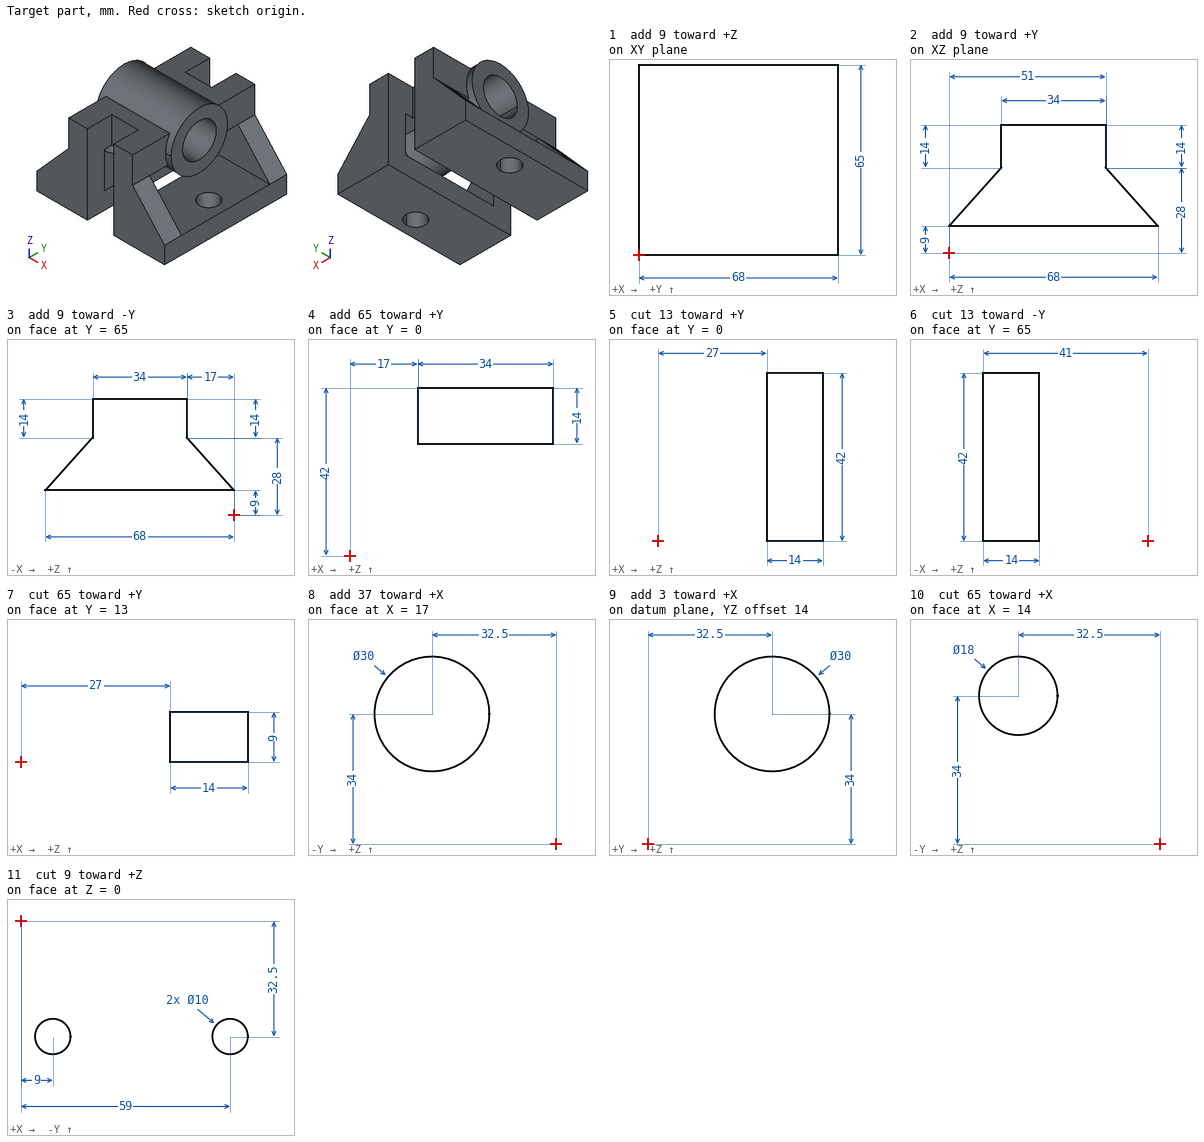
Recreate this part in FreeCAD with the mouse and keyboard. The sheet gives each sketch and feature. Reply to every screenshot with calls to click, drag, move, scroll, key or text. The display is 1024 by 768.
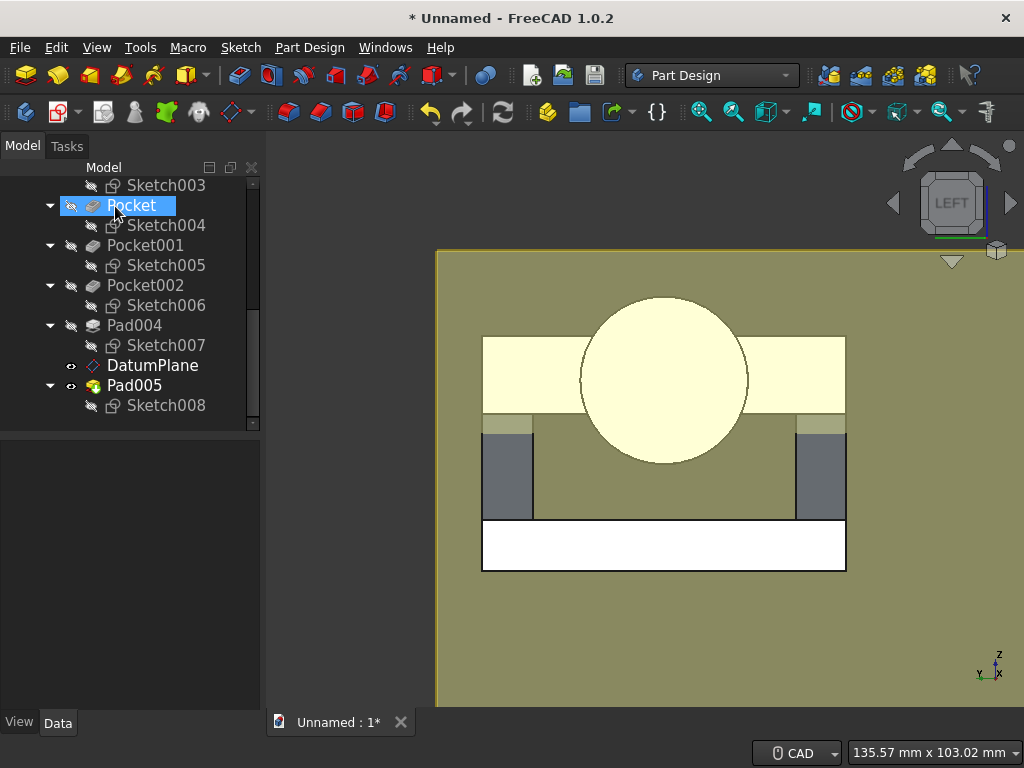
click(116, 366)
key(space)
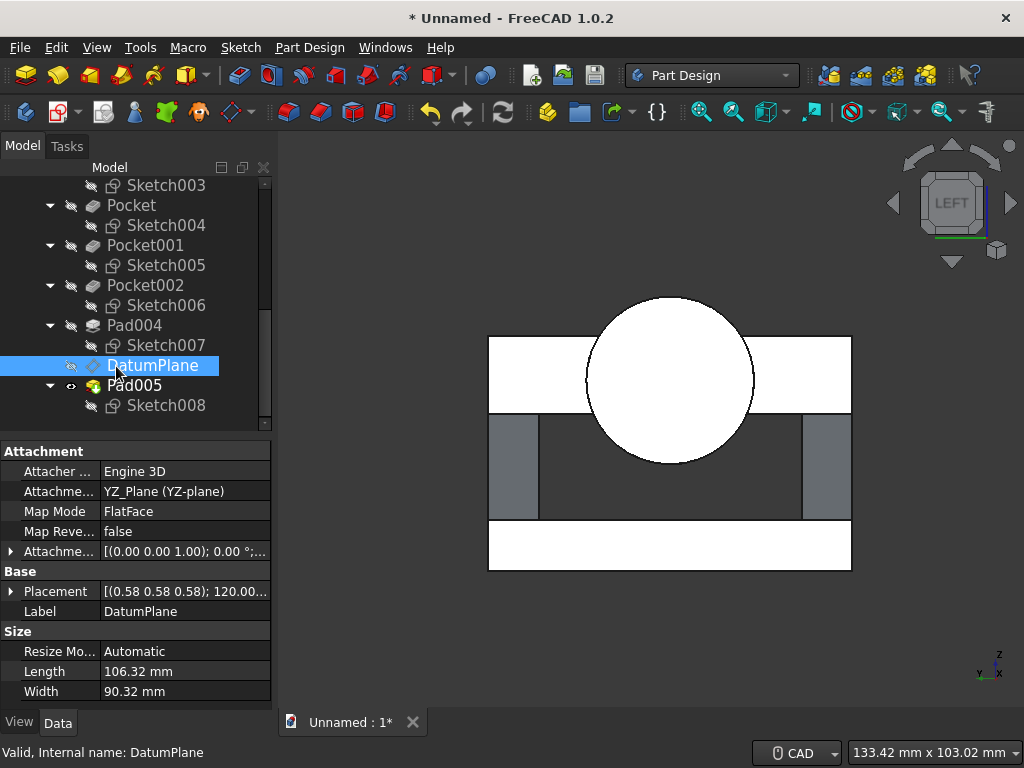
click(670, 379)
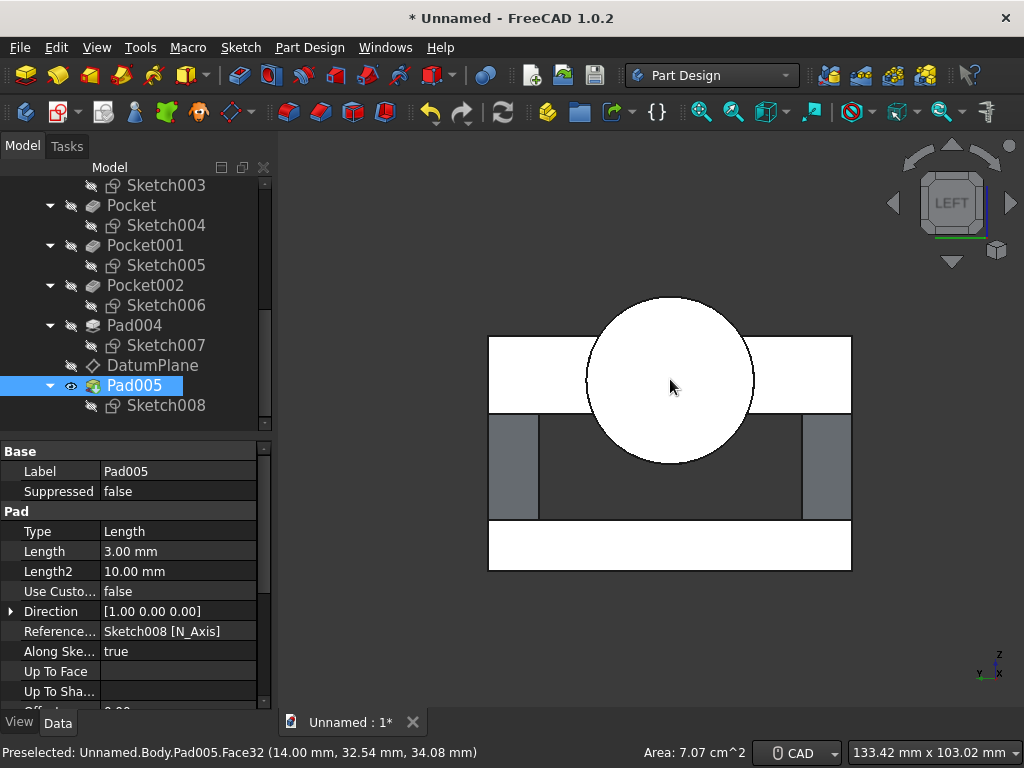
click(58, 112)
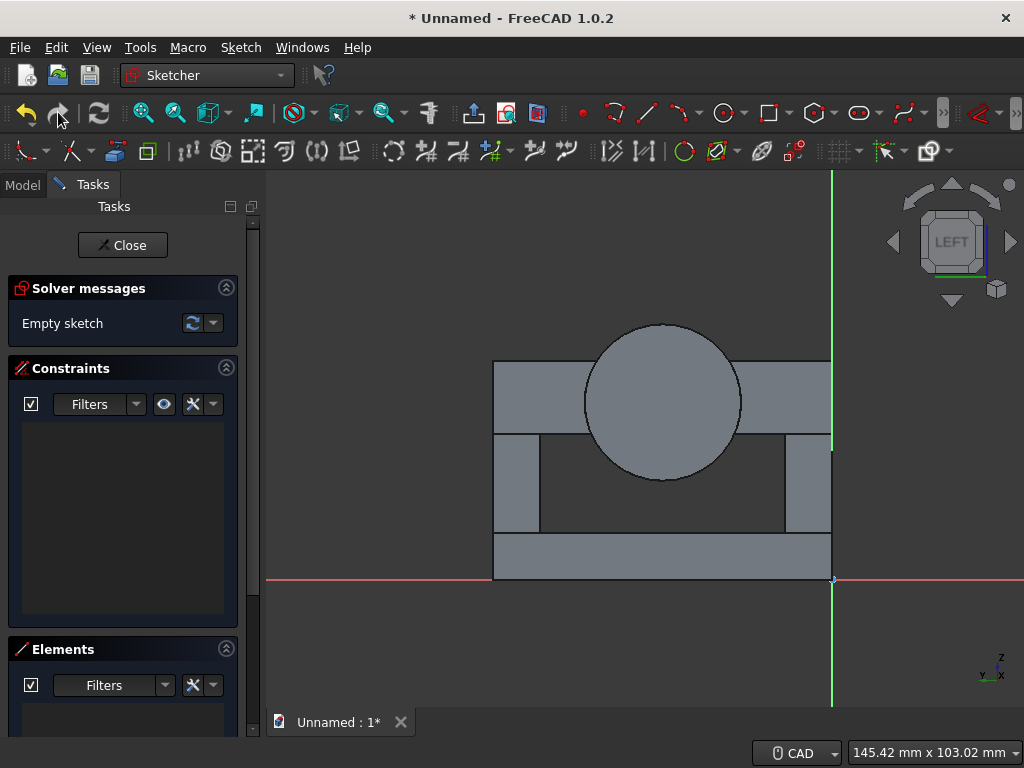
key(q)
key(s)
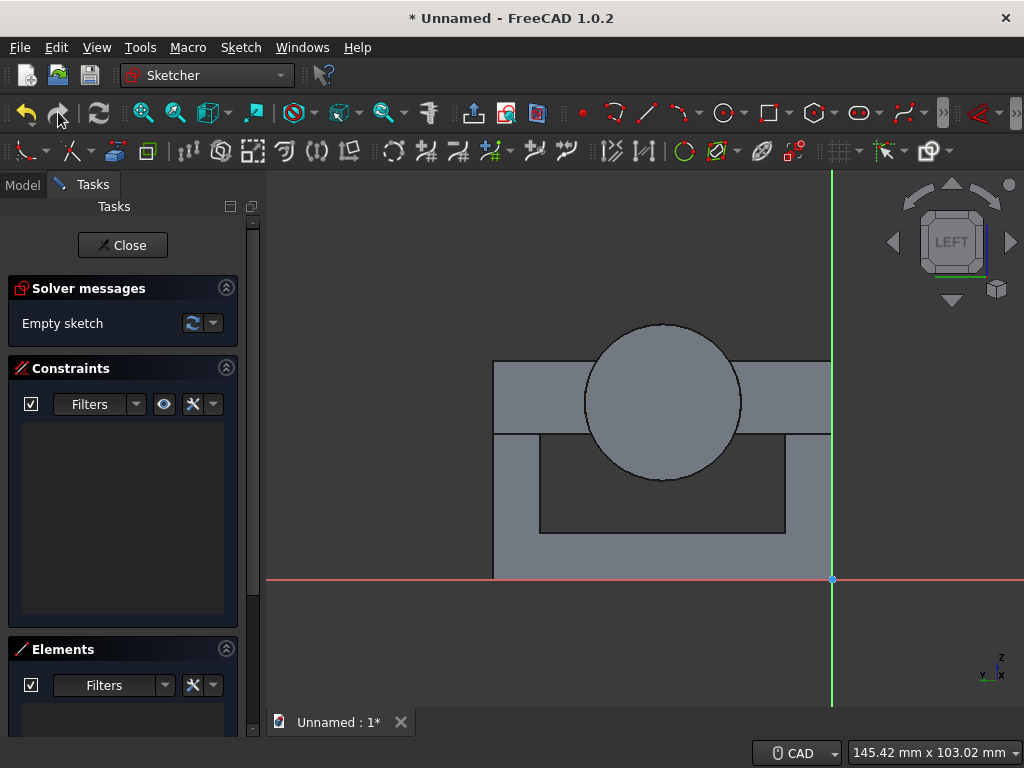
scroll(859, 527, up, 2)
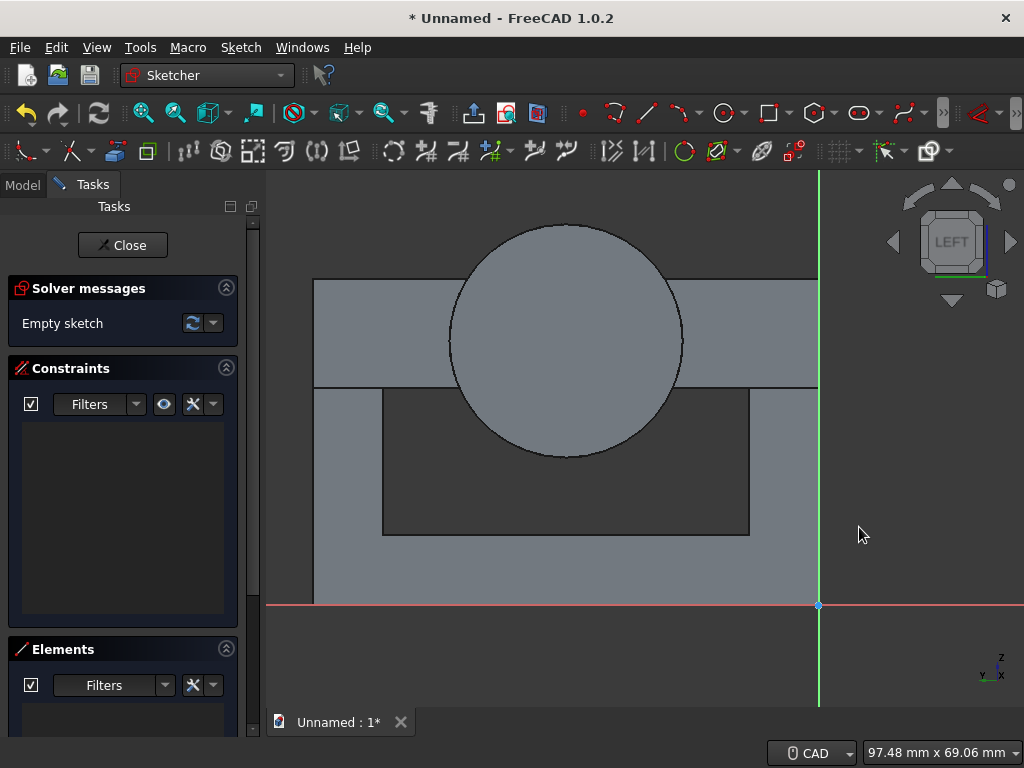
click(724, 114)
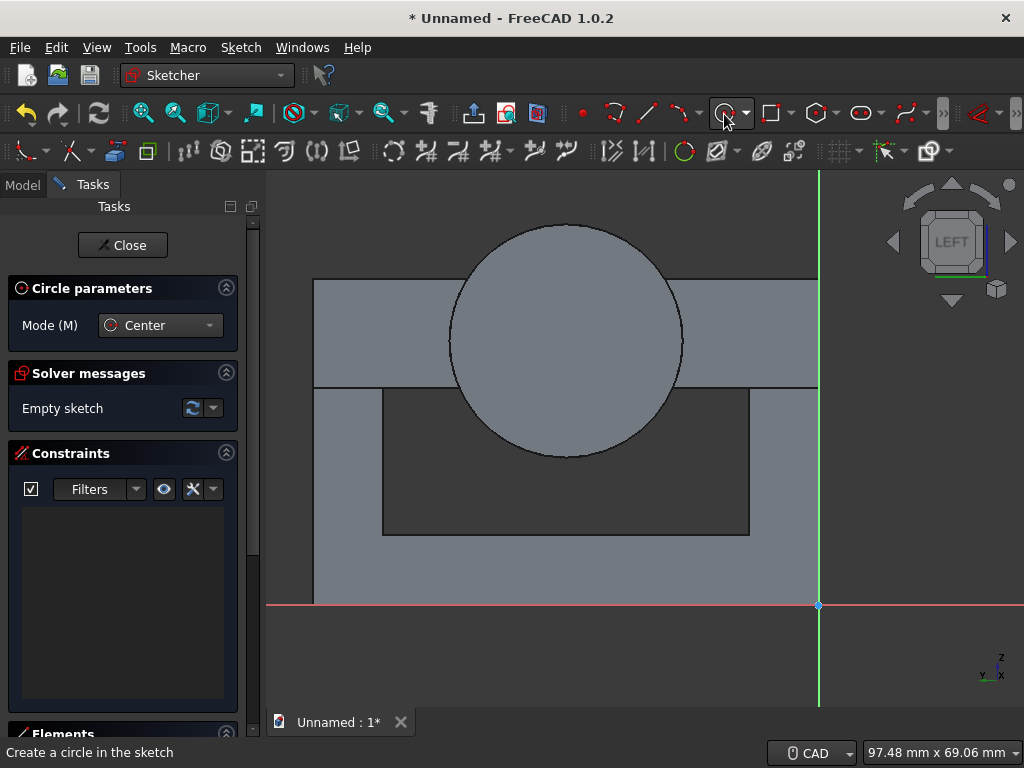
click(566, 341)
move(616, 292)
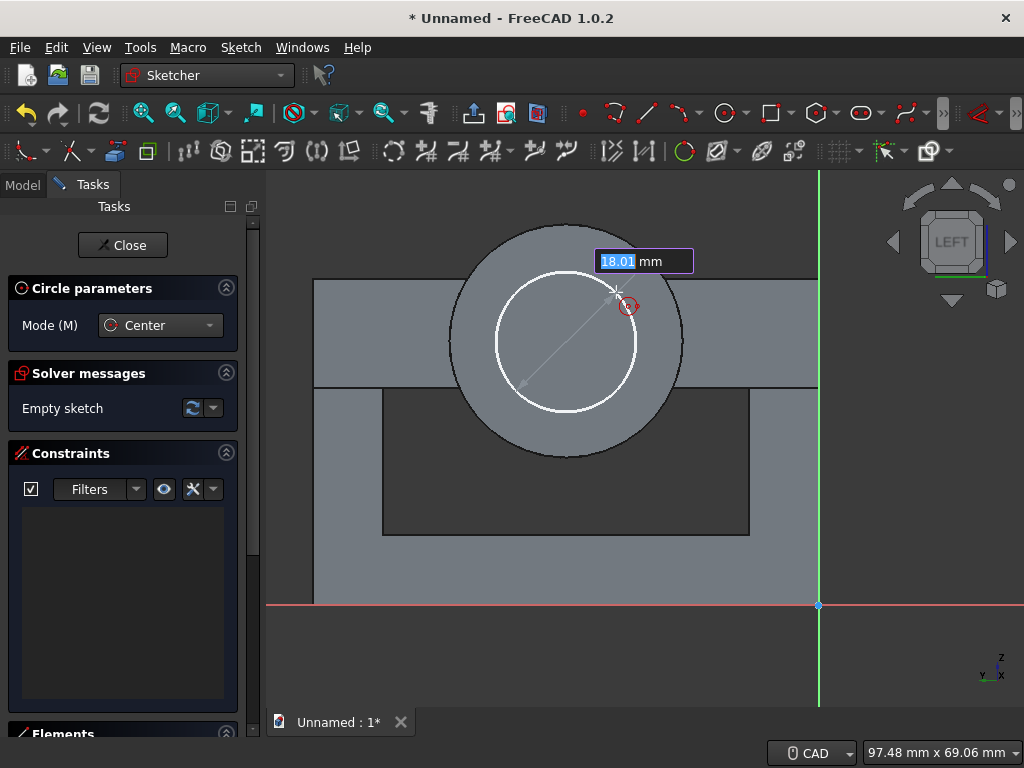
text(18)
key(Return)
key(Escape)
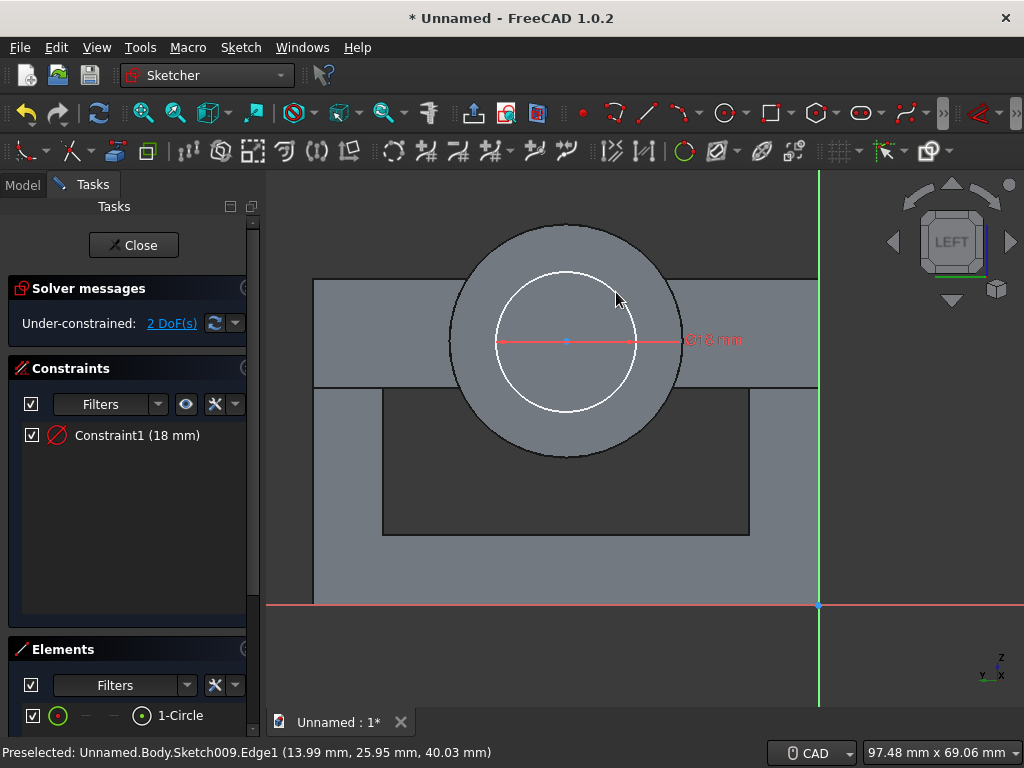
key(d)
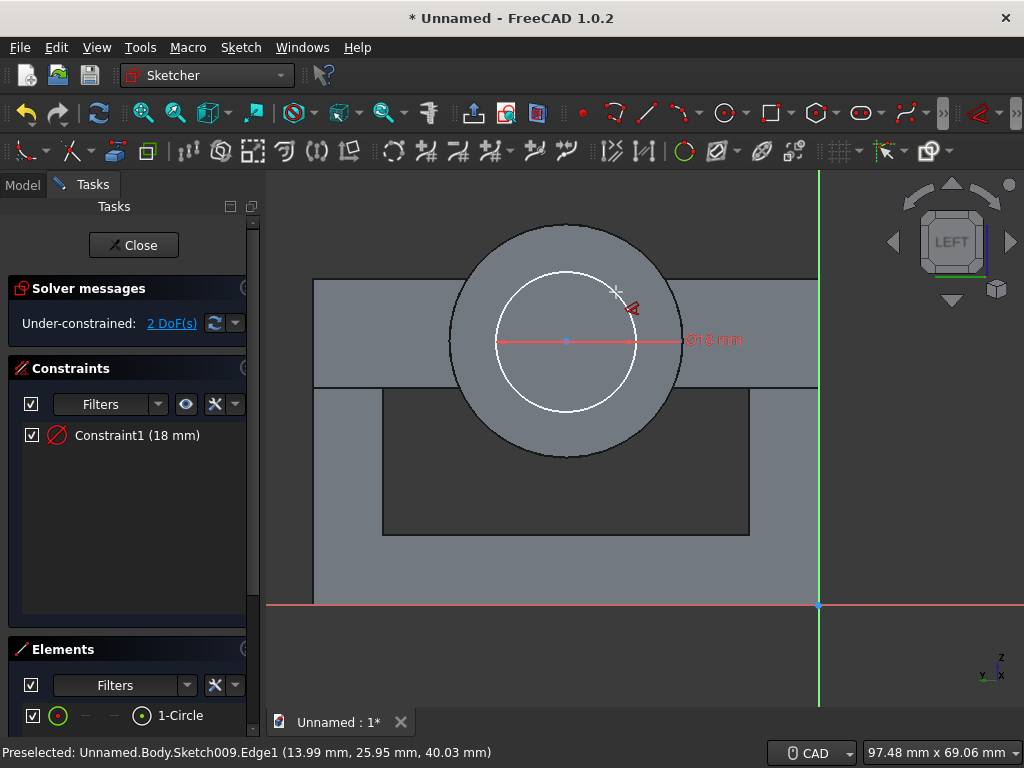
click(566, 342)
click(853, 474)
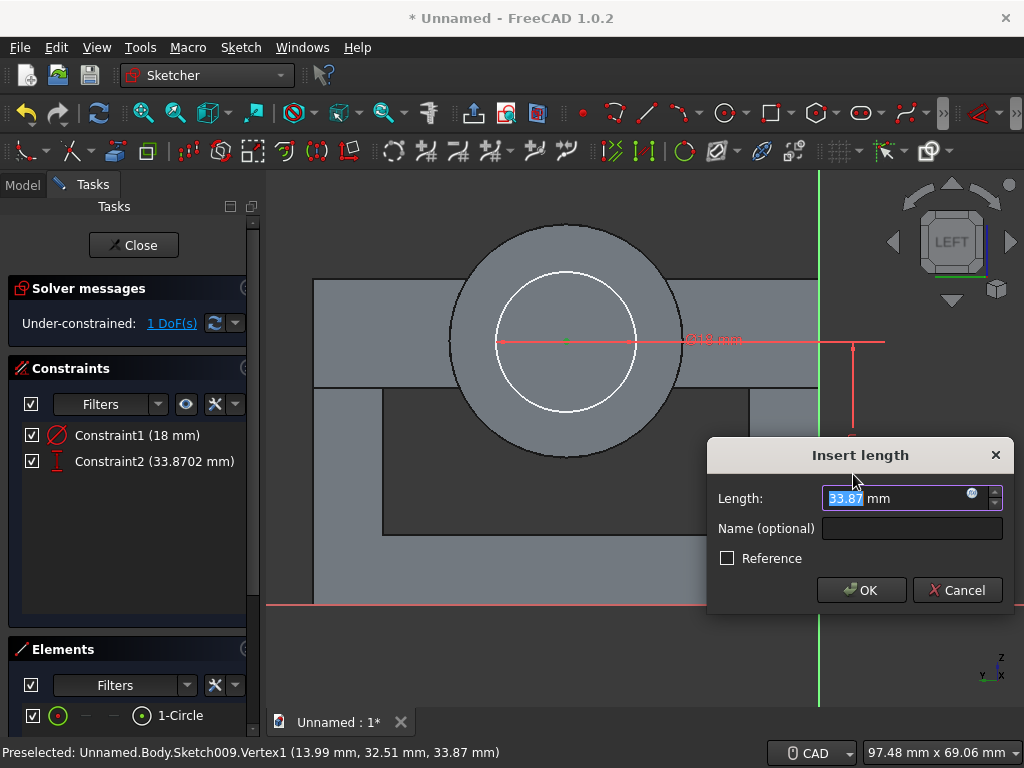
text(34)
key(Return)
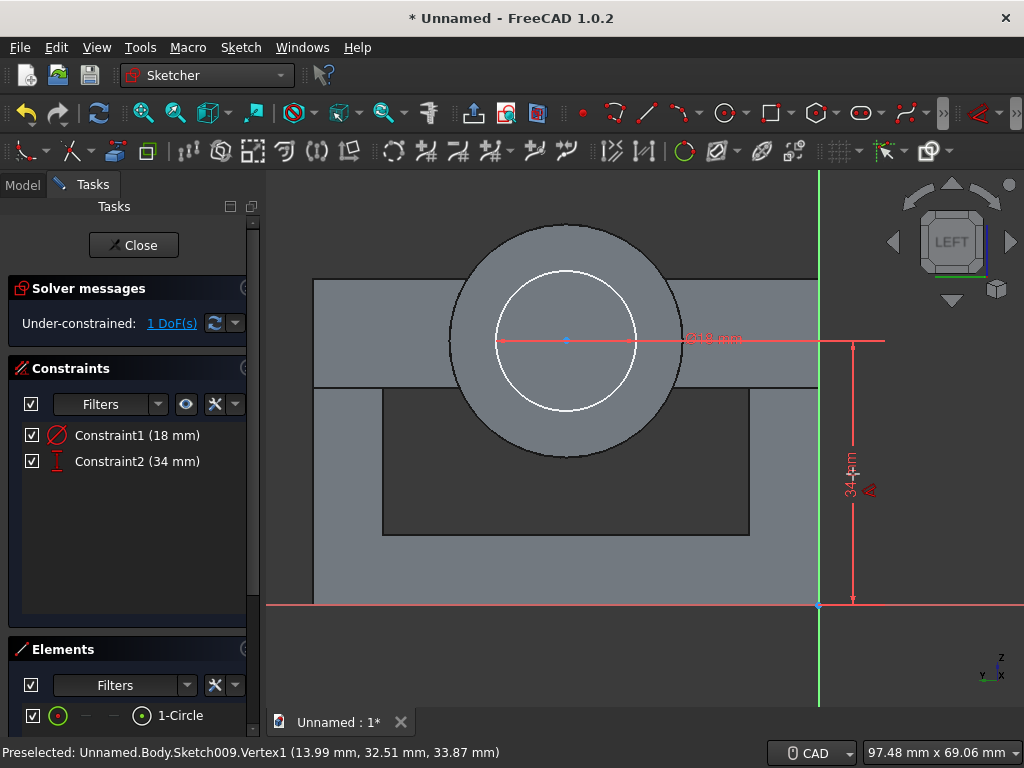
click(566, 341)
click(692, 639)